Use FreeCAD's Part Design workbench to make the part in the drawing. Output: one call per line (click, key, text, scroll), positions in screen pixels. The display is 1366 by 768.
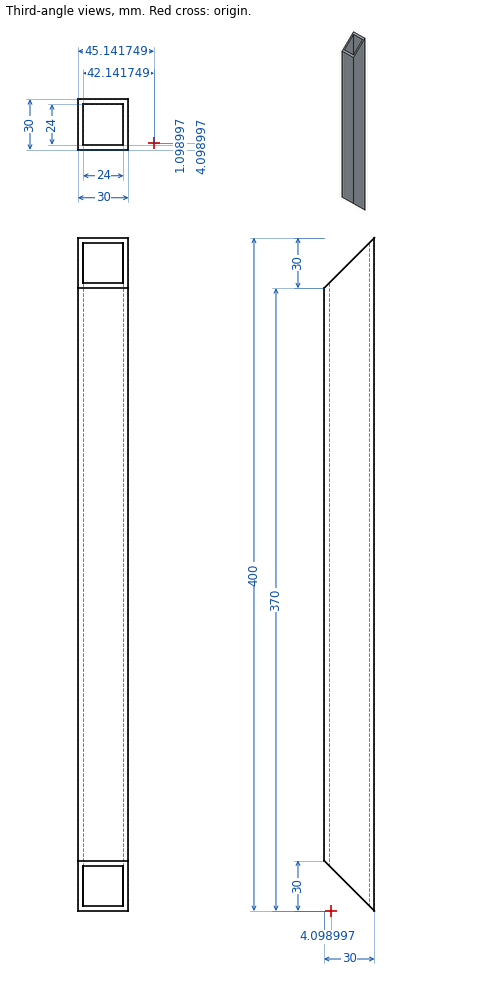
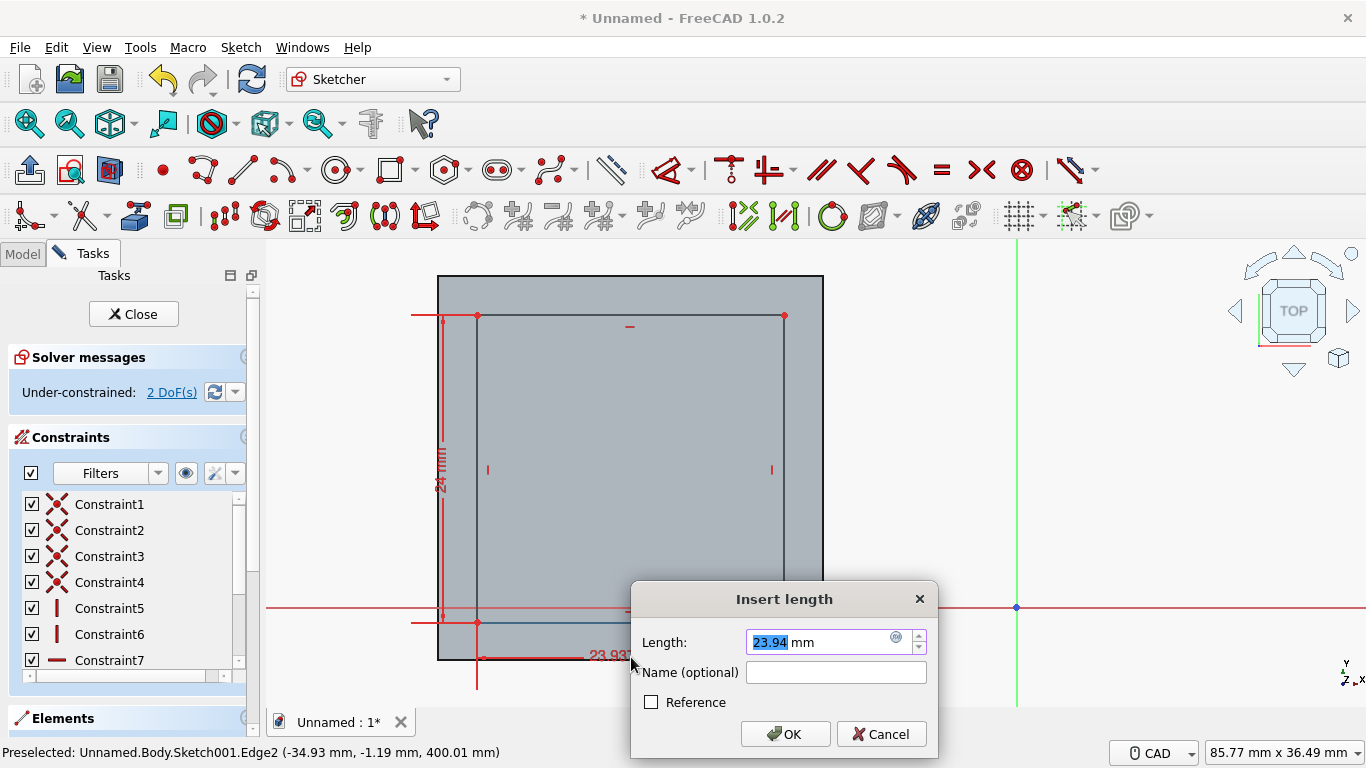
text(24)
key(Return)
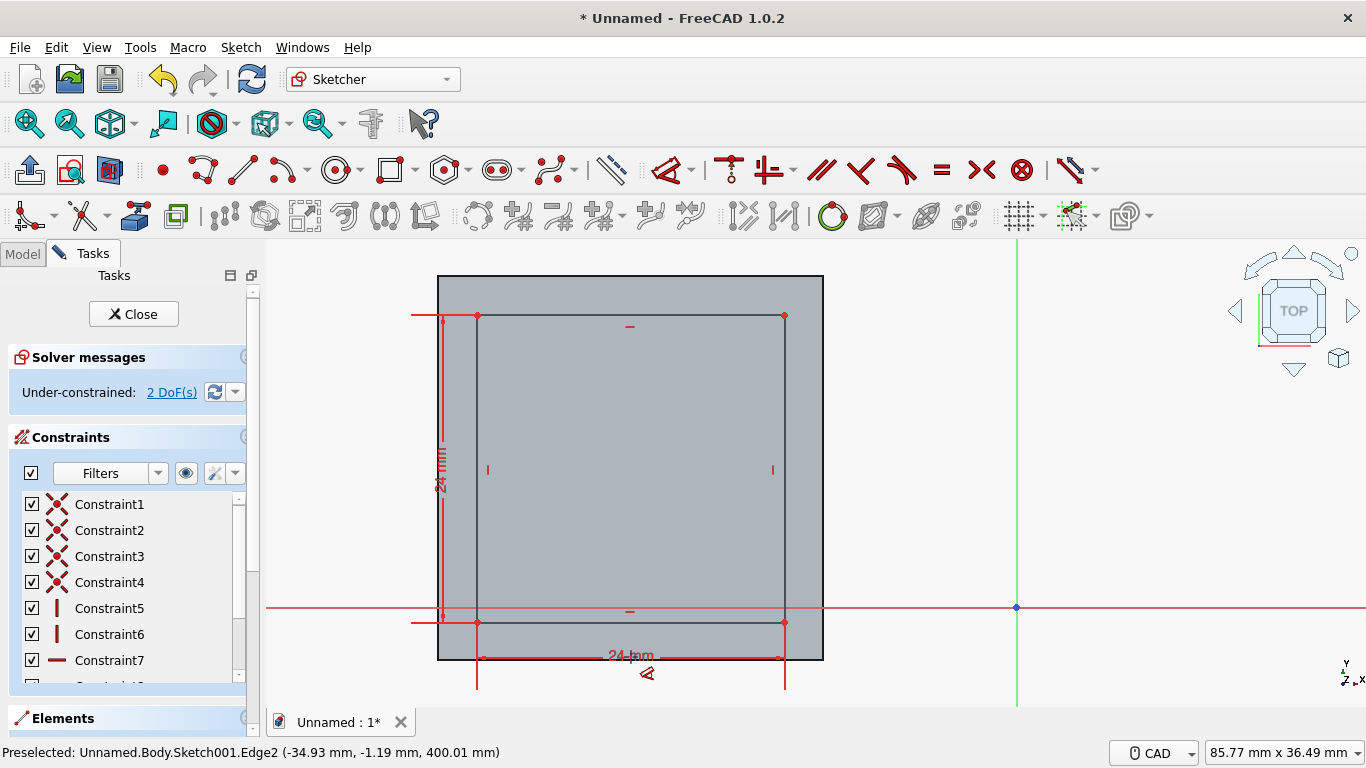
scroll(477, 623, up, 6)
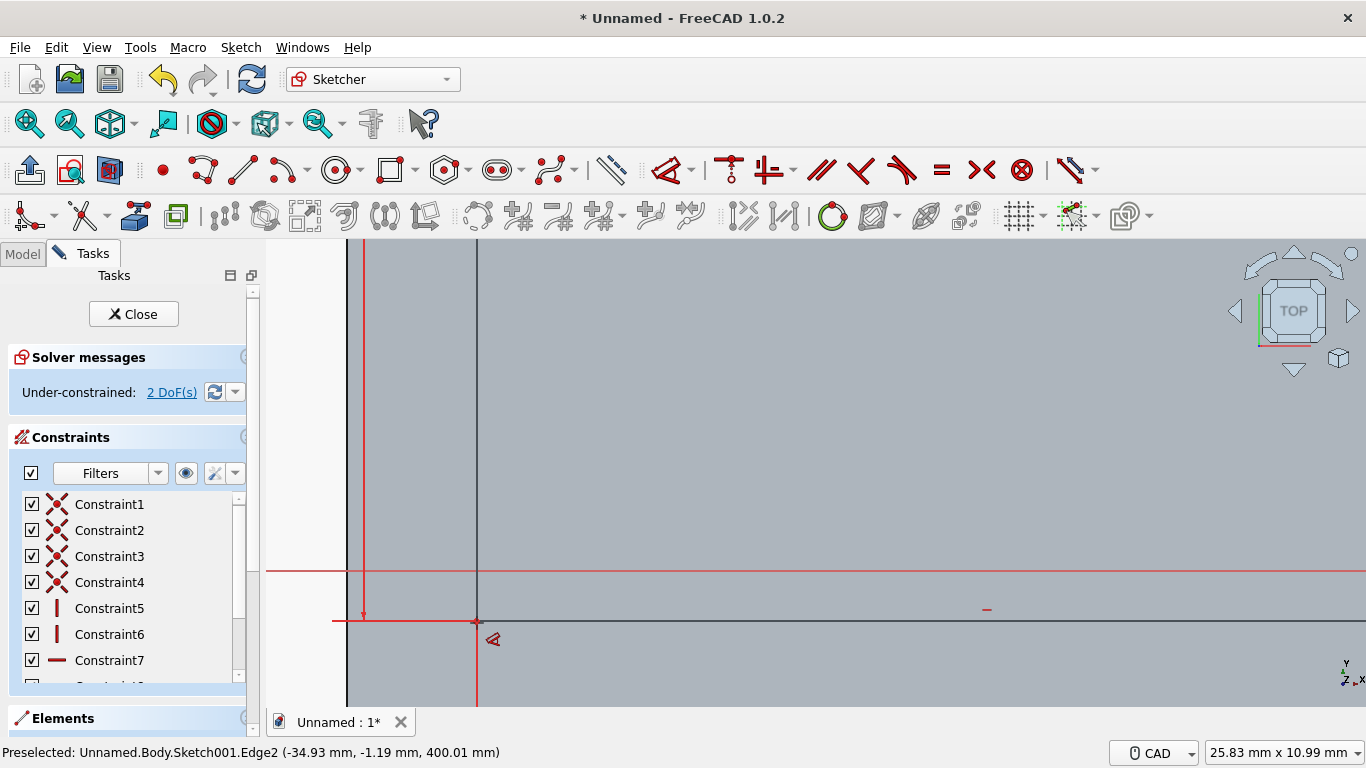
click(477, 621)
click(443, 596)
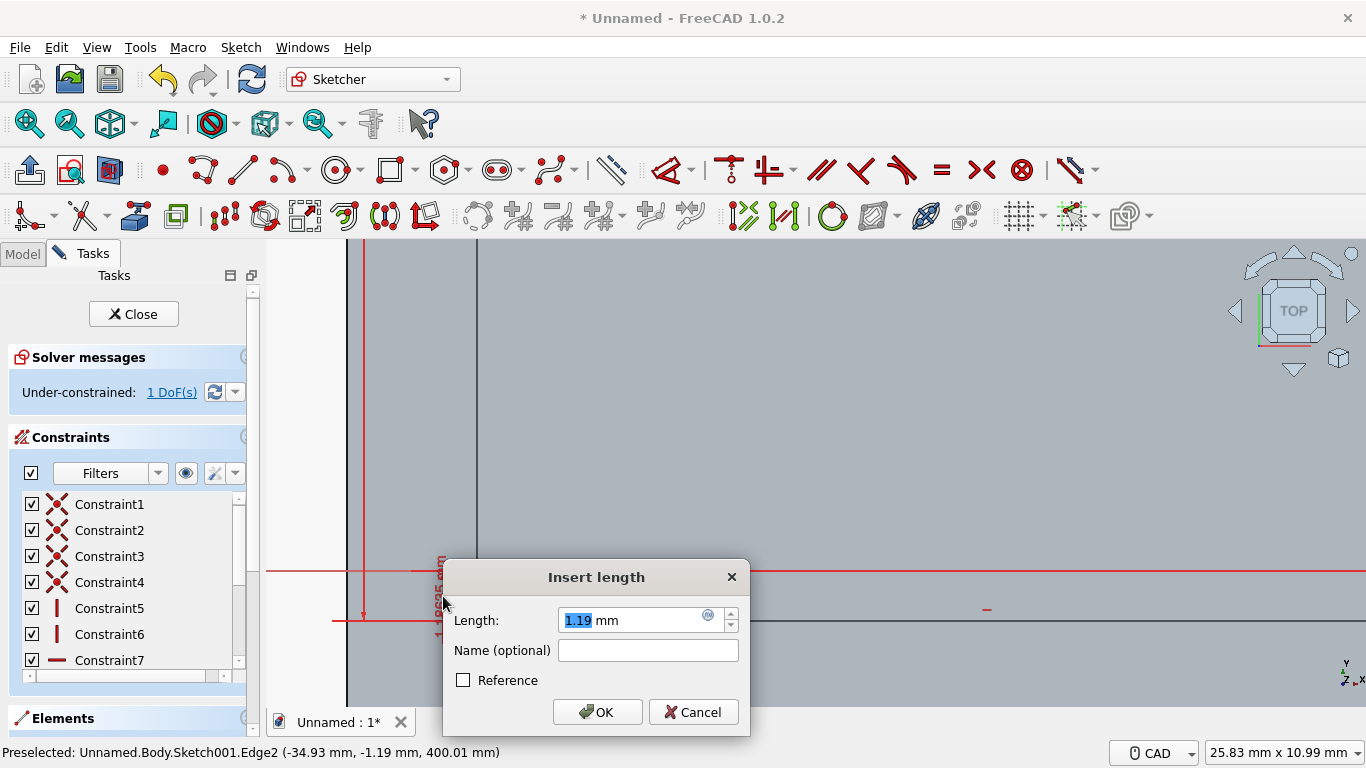
text(1.098997)
key(Return)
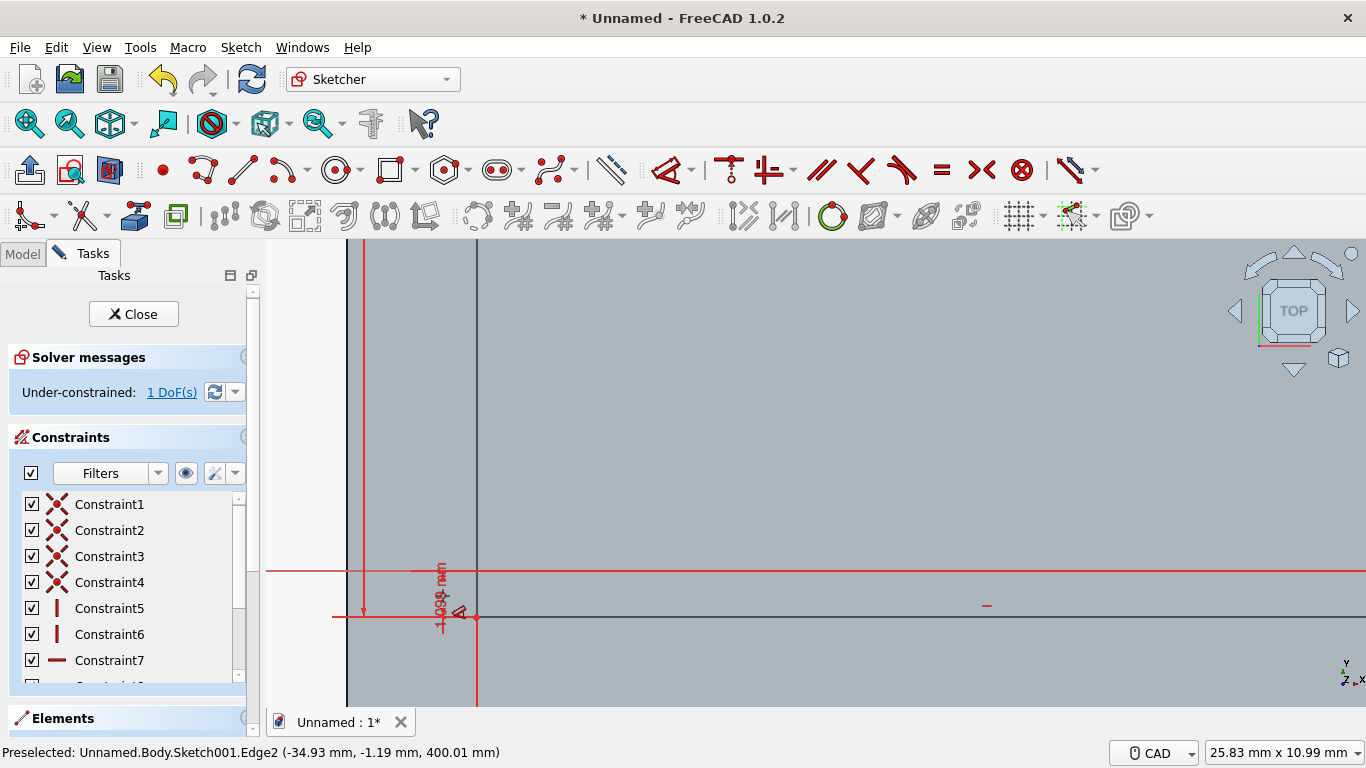
scroll(478, 631, down, 6)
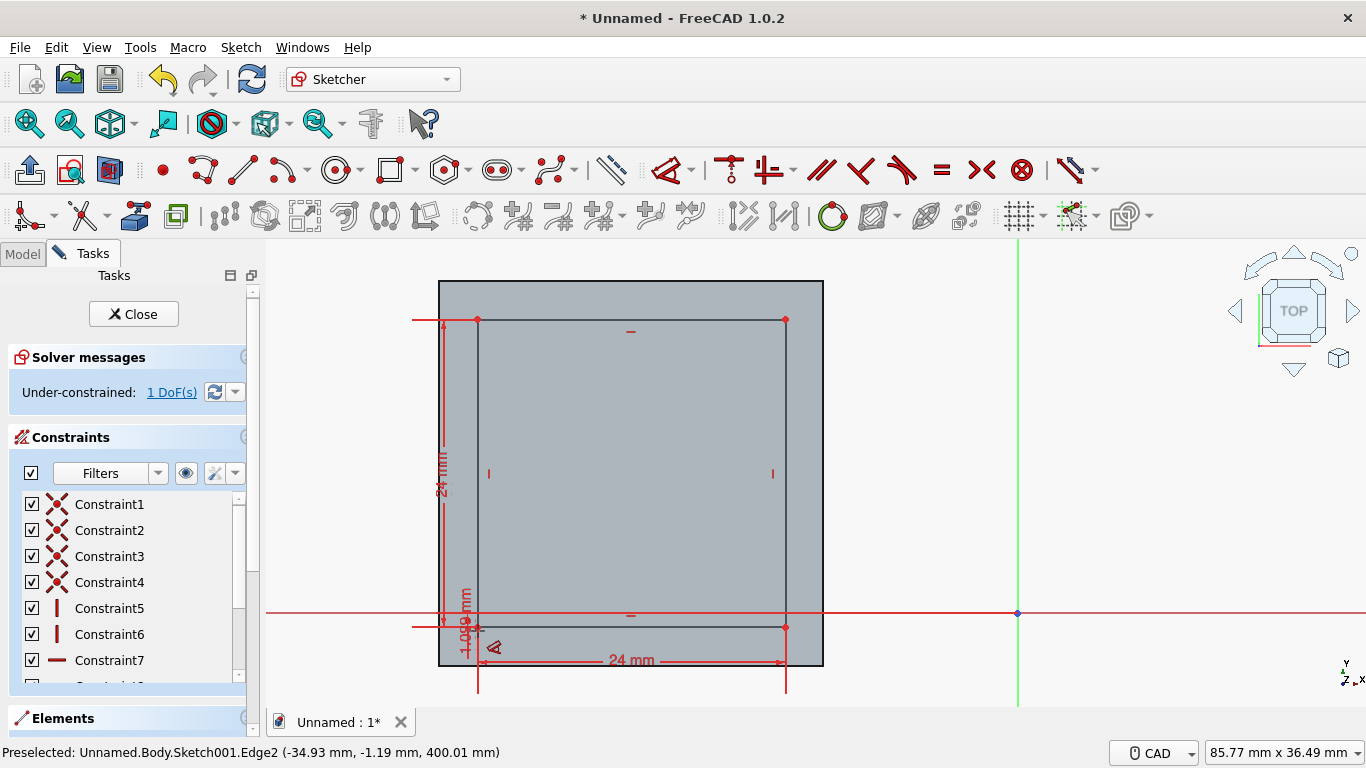
click(478, 320)
click(748, 286)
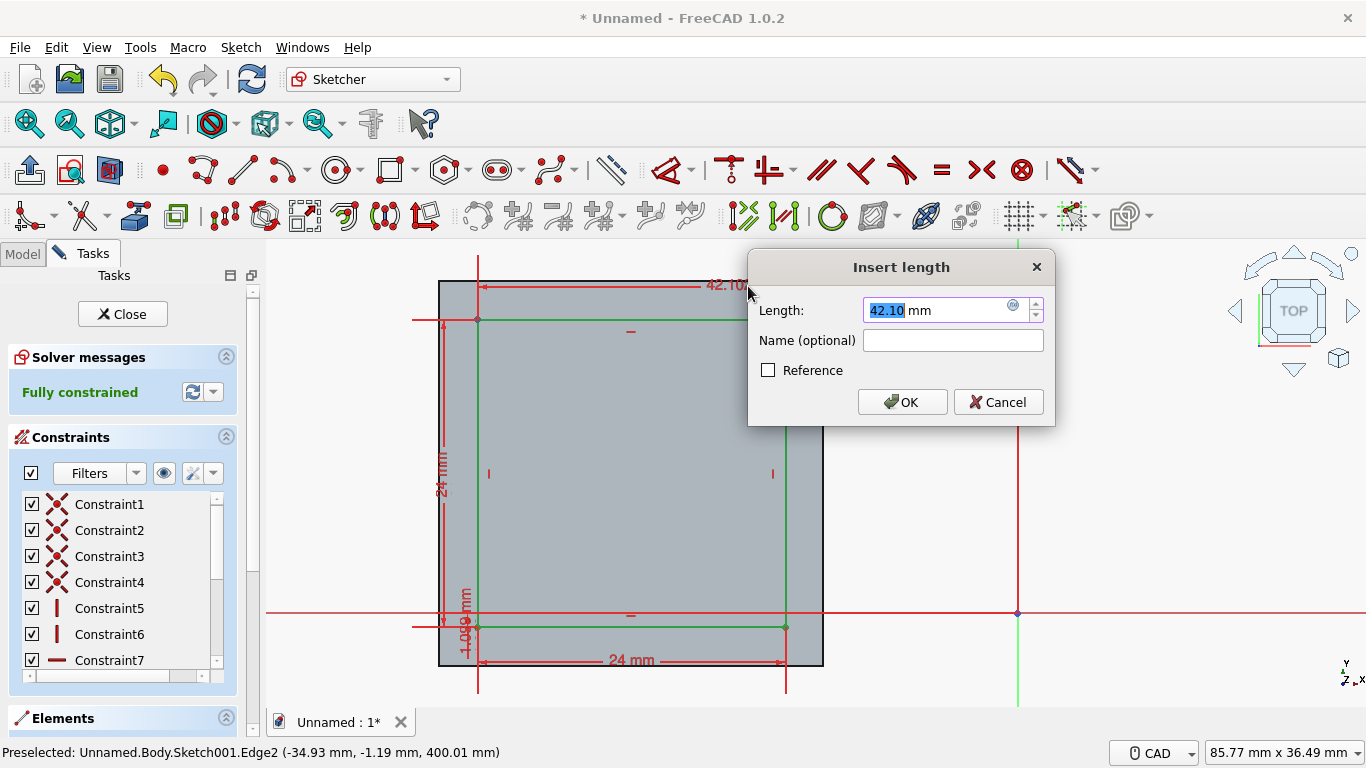
text(42.141749)
key(Return)
key(Escape)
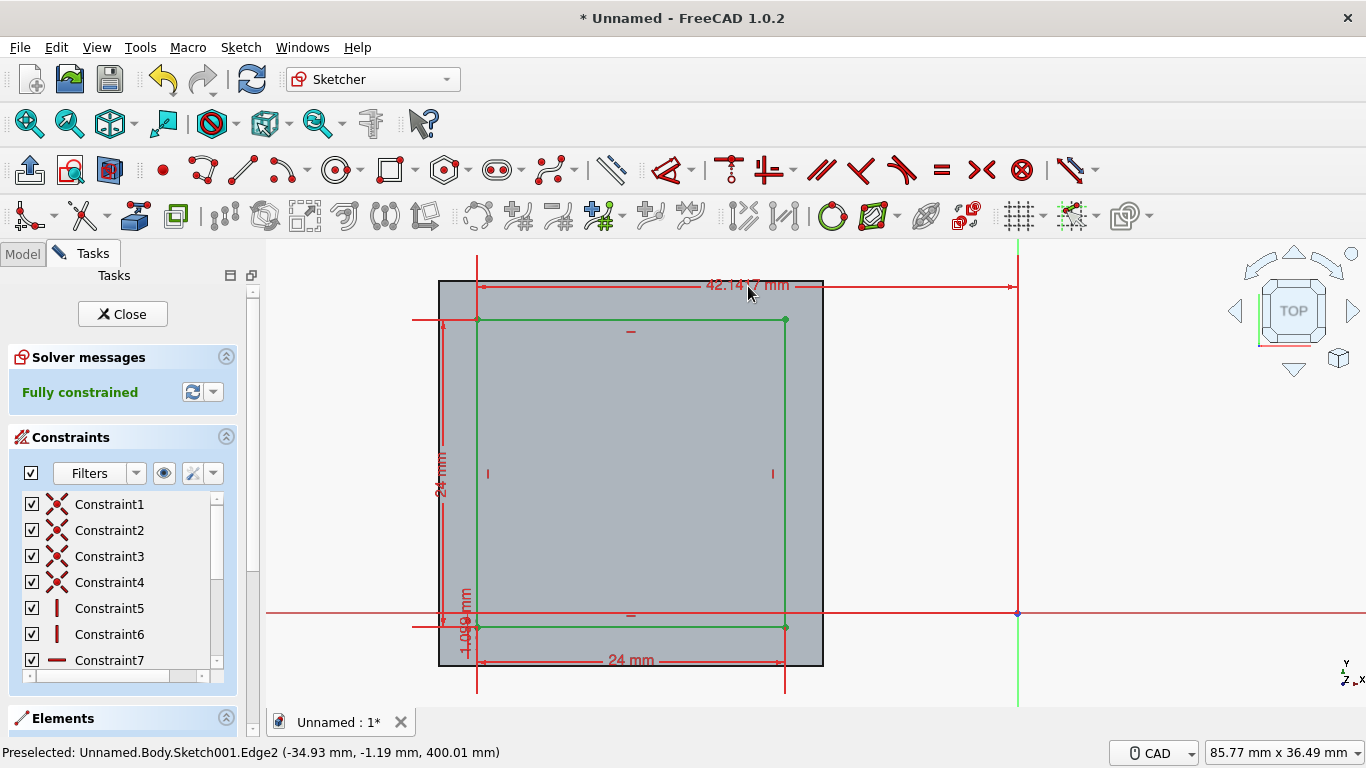
click(123, 314)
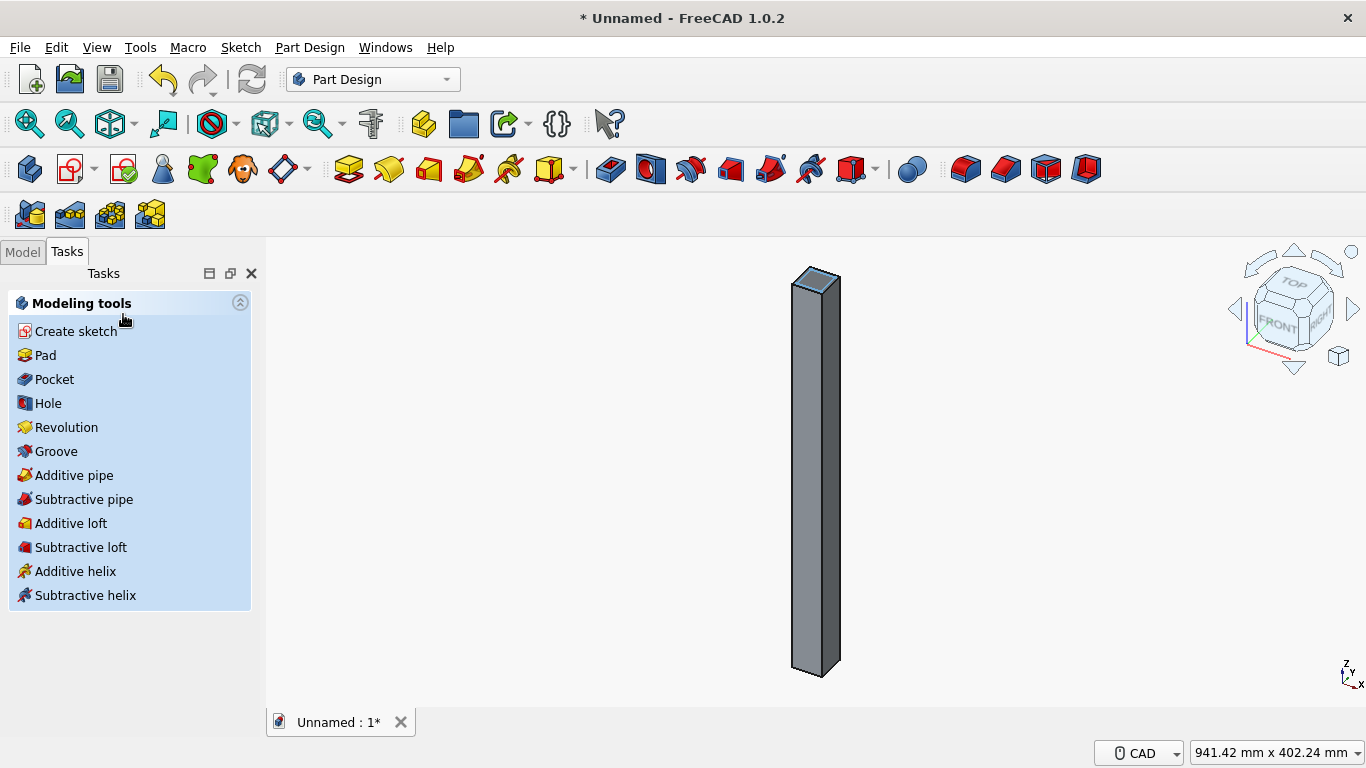
click(612, 170)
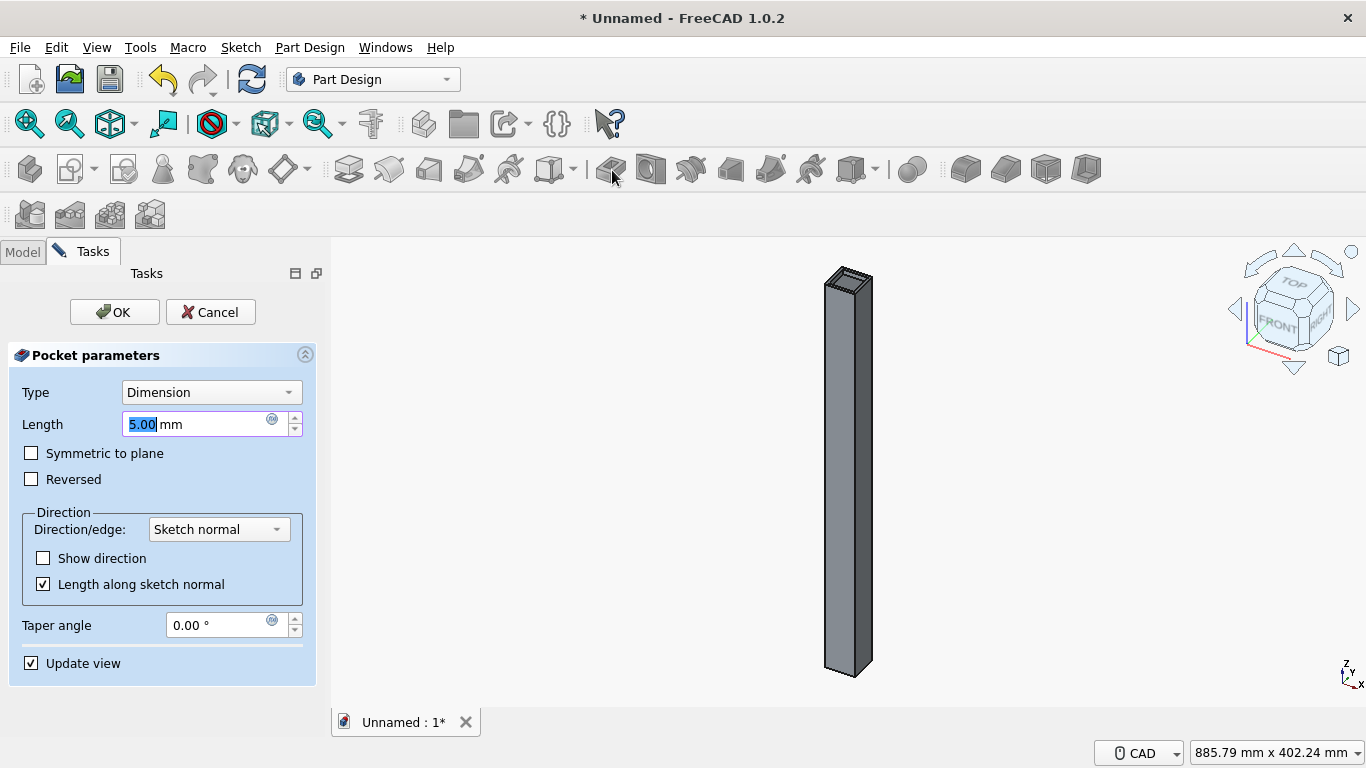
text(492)
key(Tab)